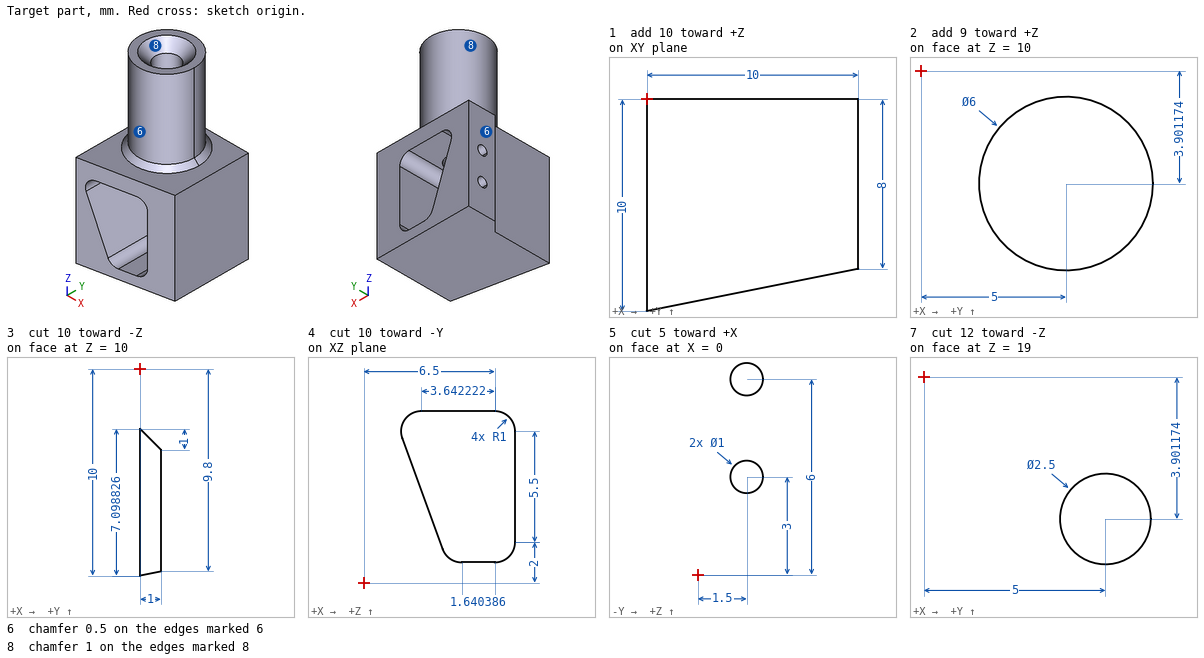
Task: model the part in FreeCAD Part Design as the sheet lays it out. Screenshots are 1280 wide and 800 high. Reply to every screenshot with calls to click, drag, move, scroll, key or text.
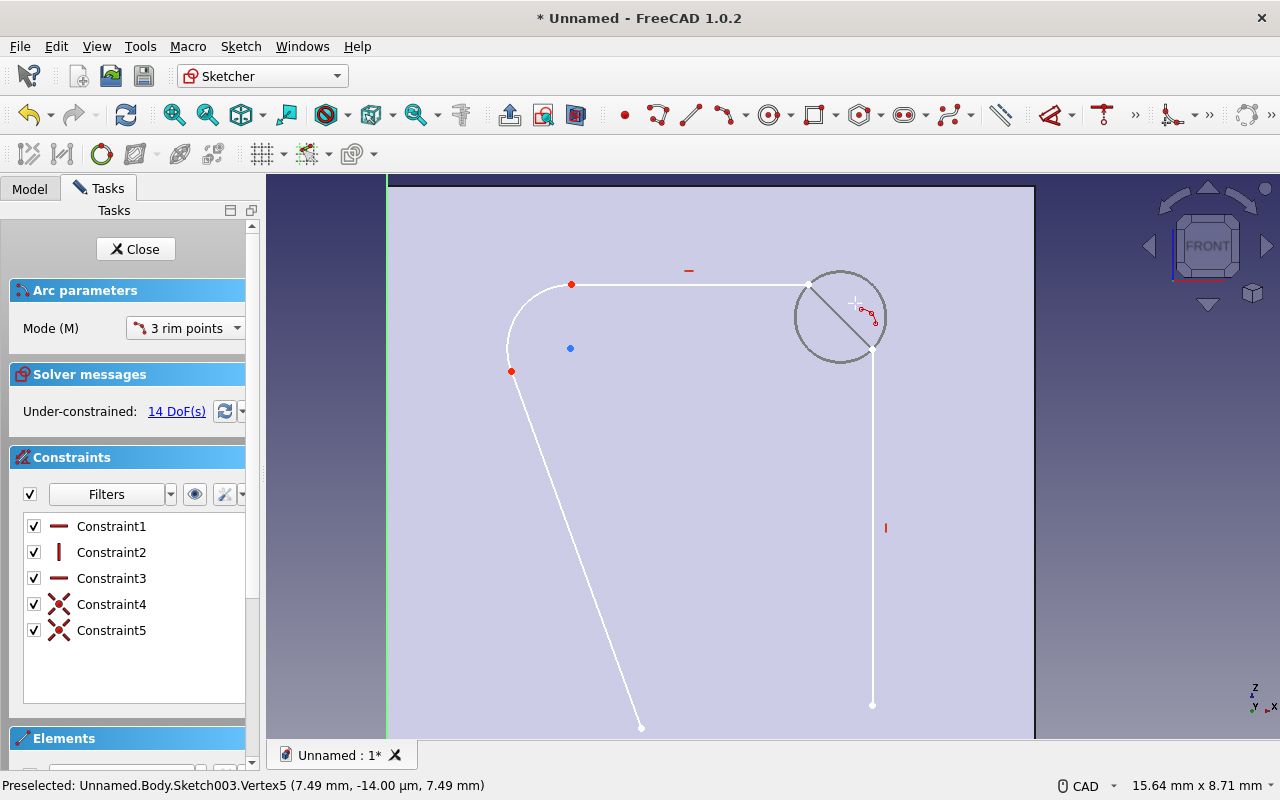
click(854, 302)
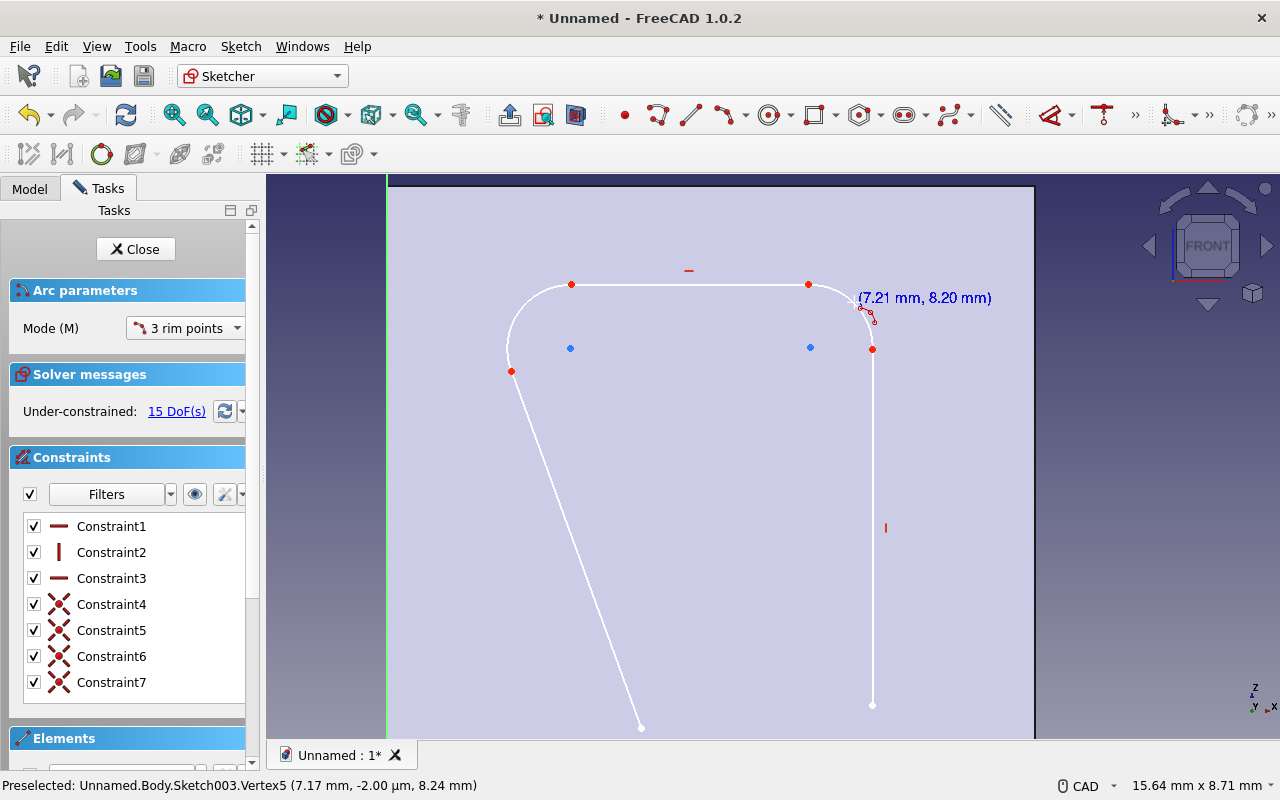
click(873, 706)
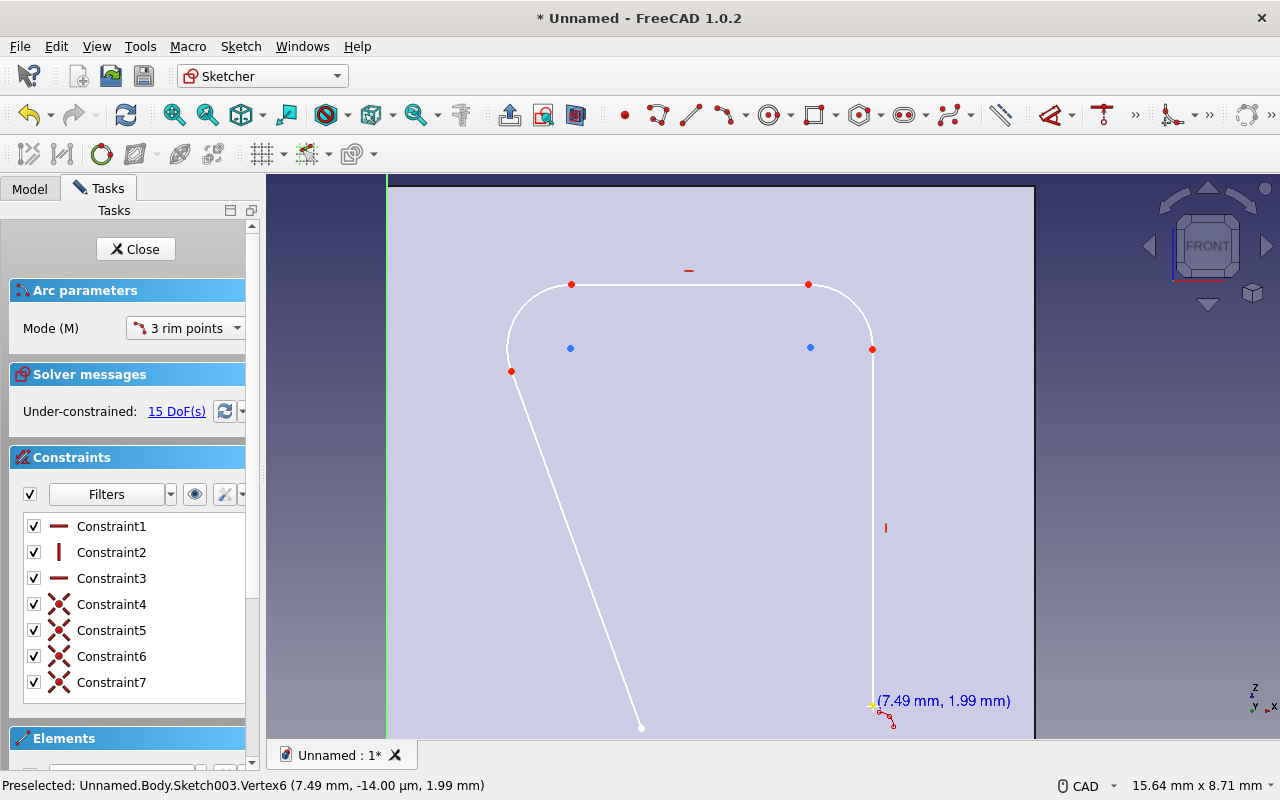
scroll(856, 248, down, 2)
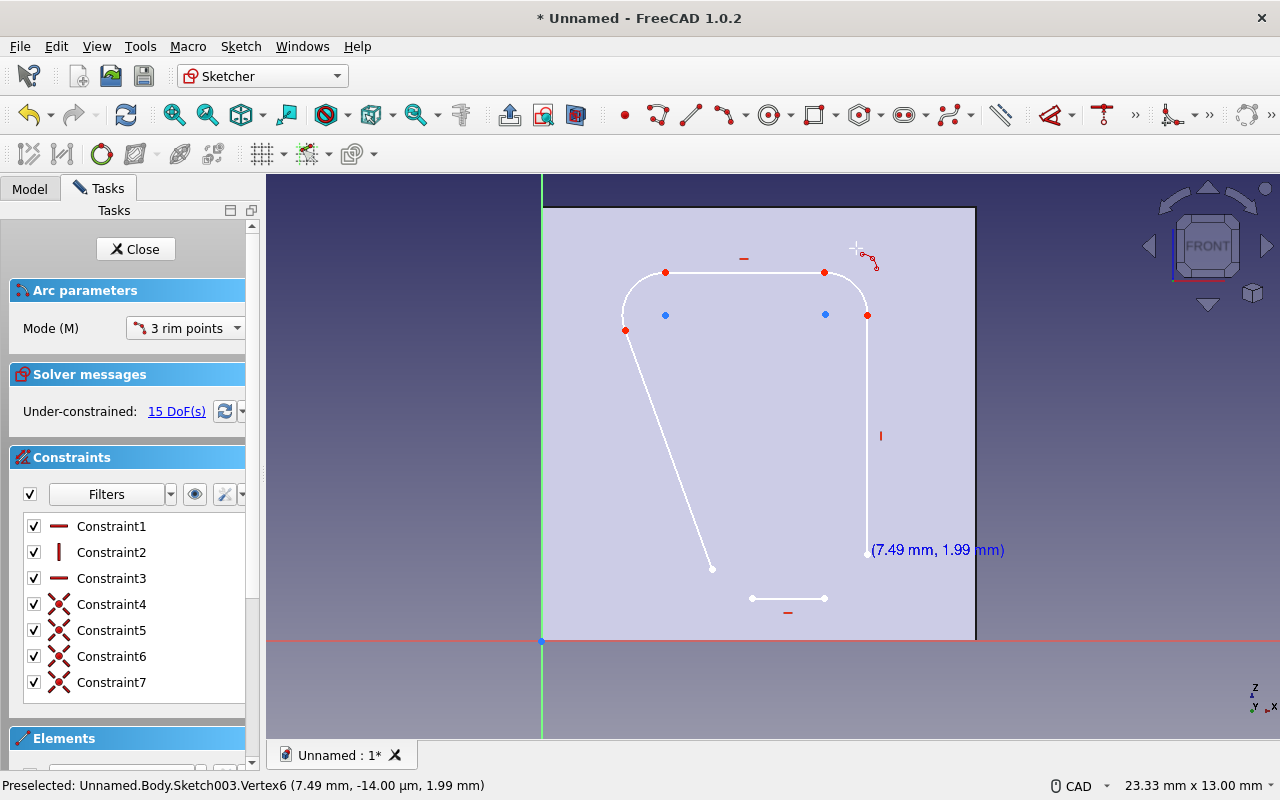
click(824, 599)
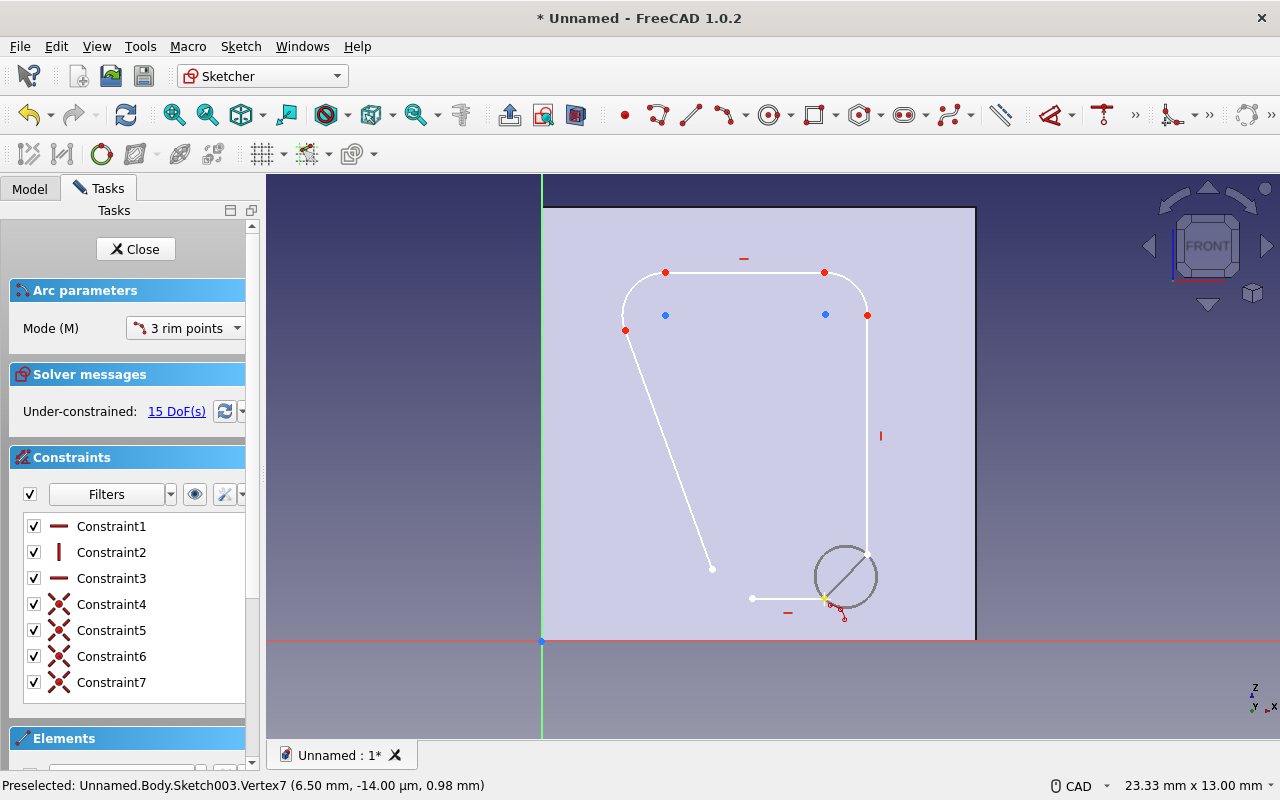
scroll(855, 585, up, 2)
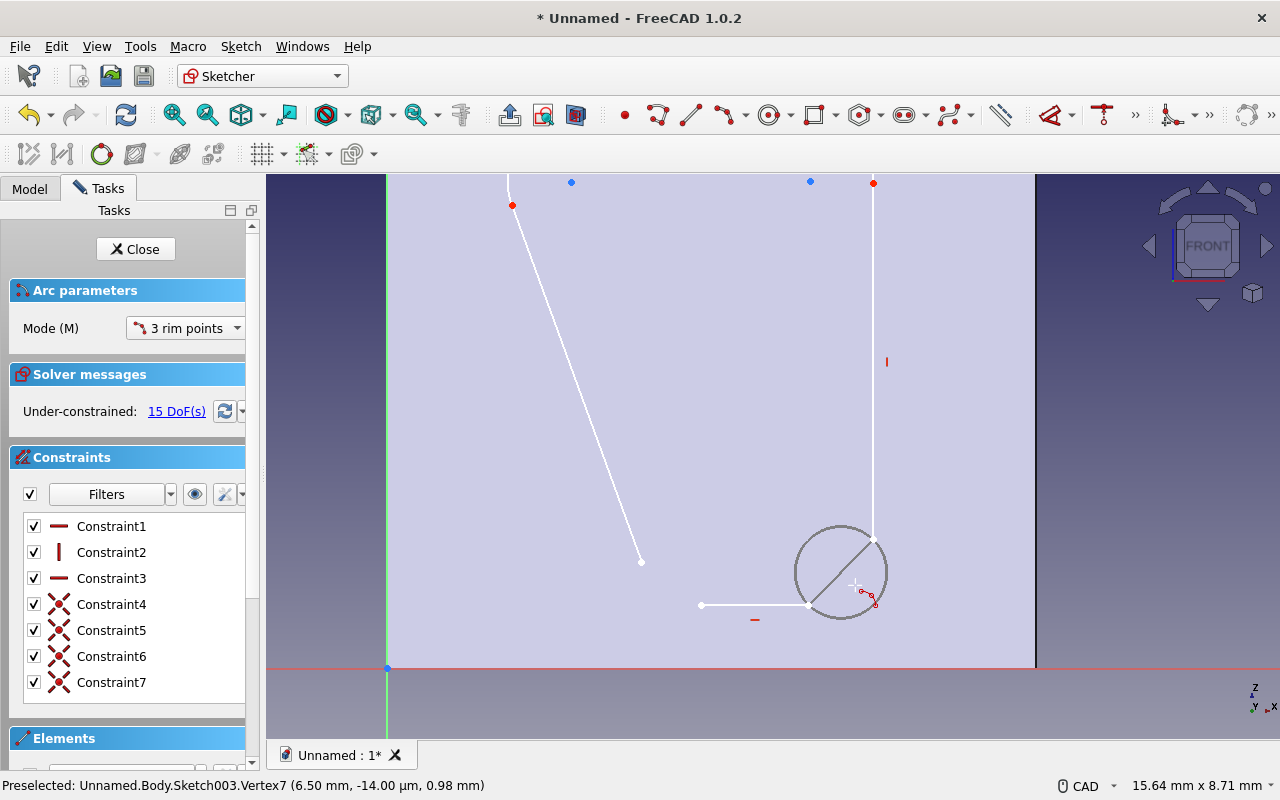
click(855, 585)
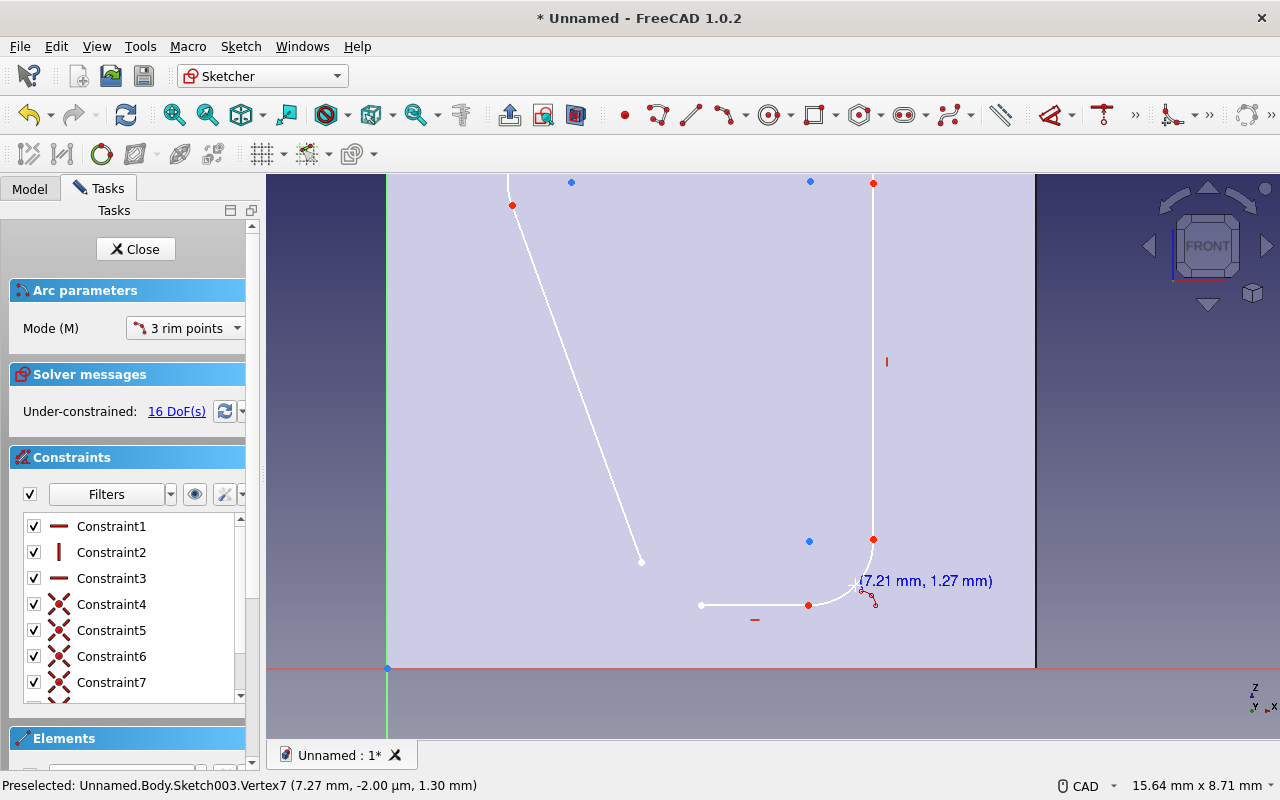
click(702, 605)
click(642, 562)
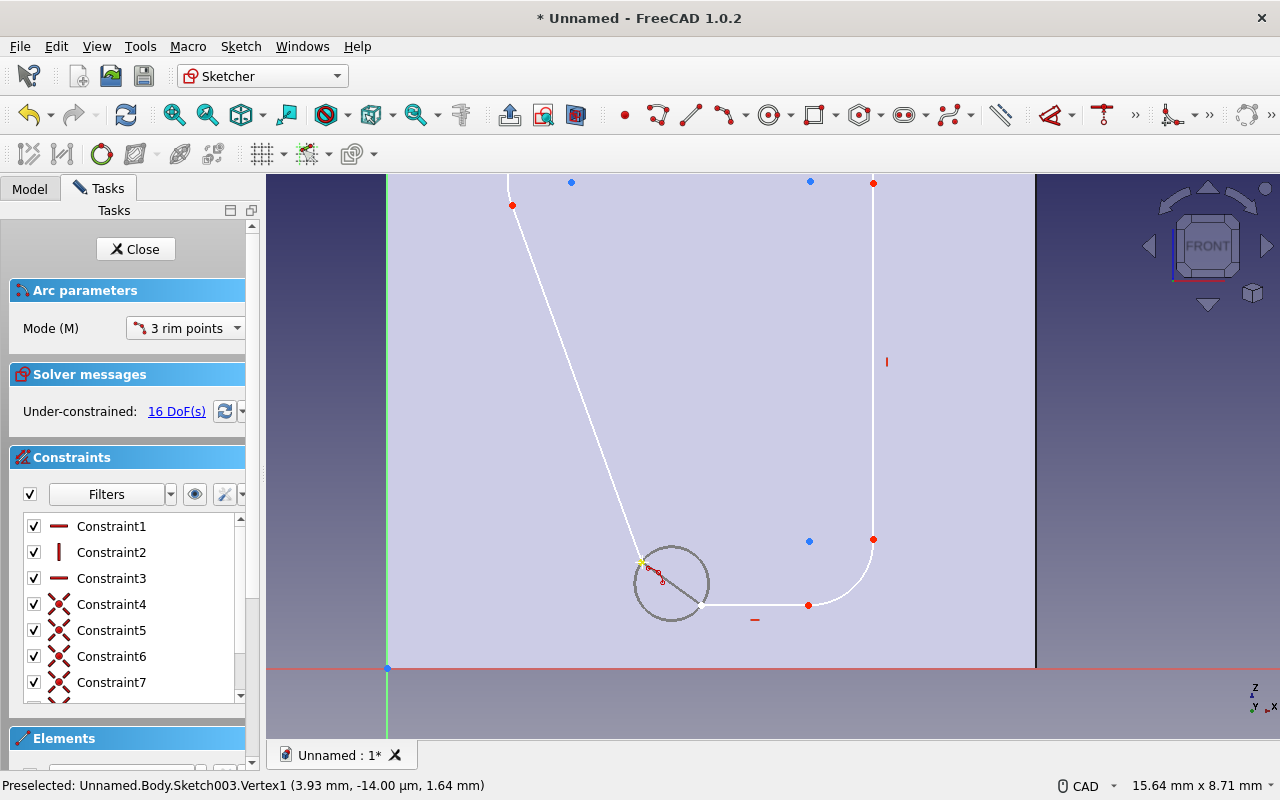
scroll(665, 592, up, 2)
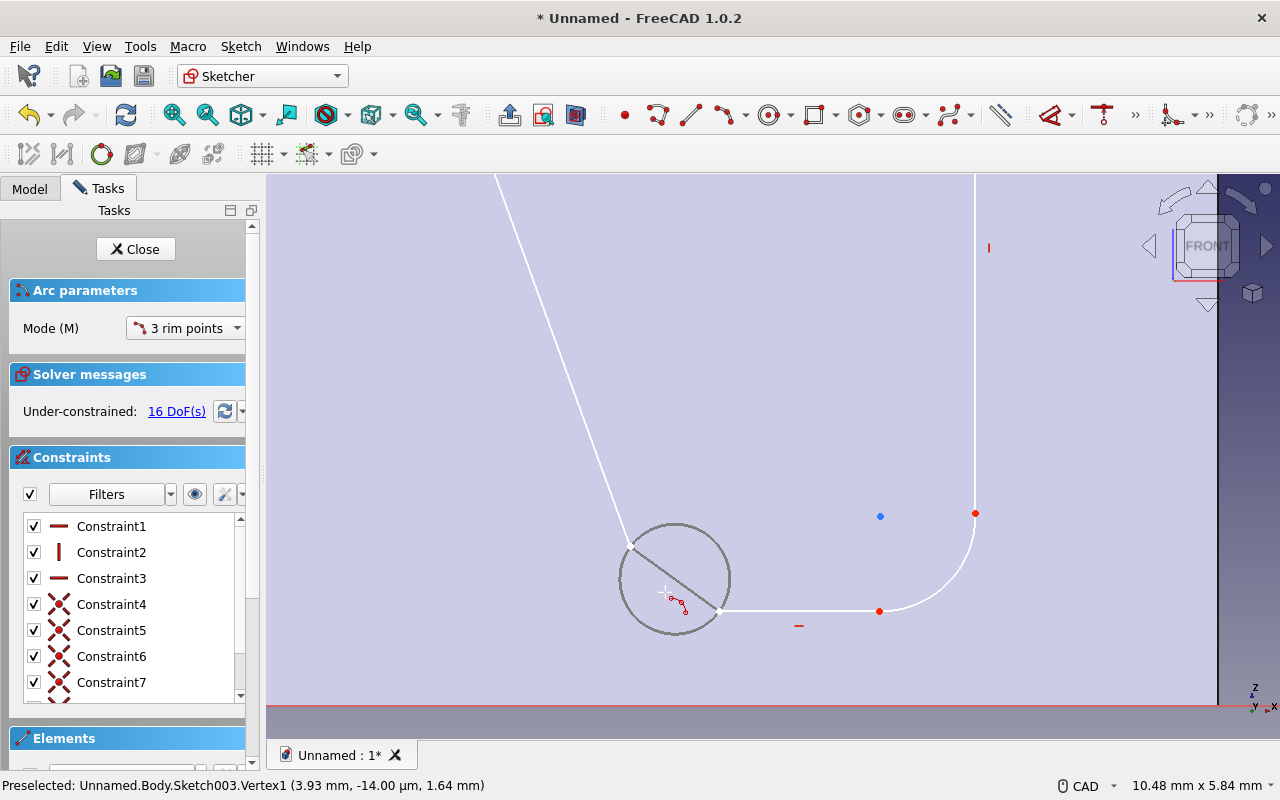
click(665, 592)
key(Escape)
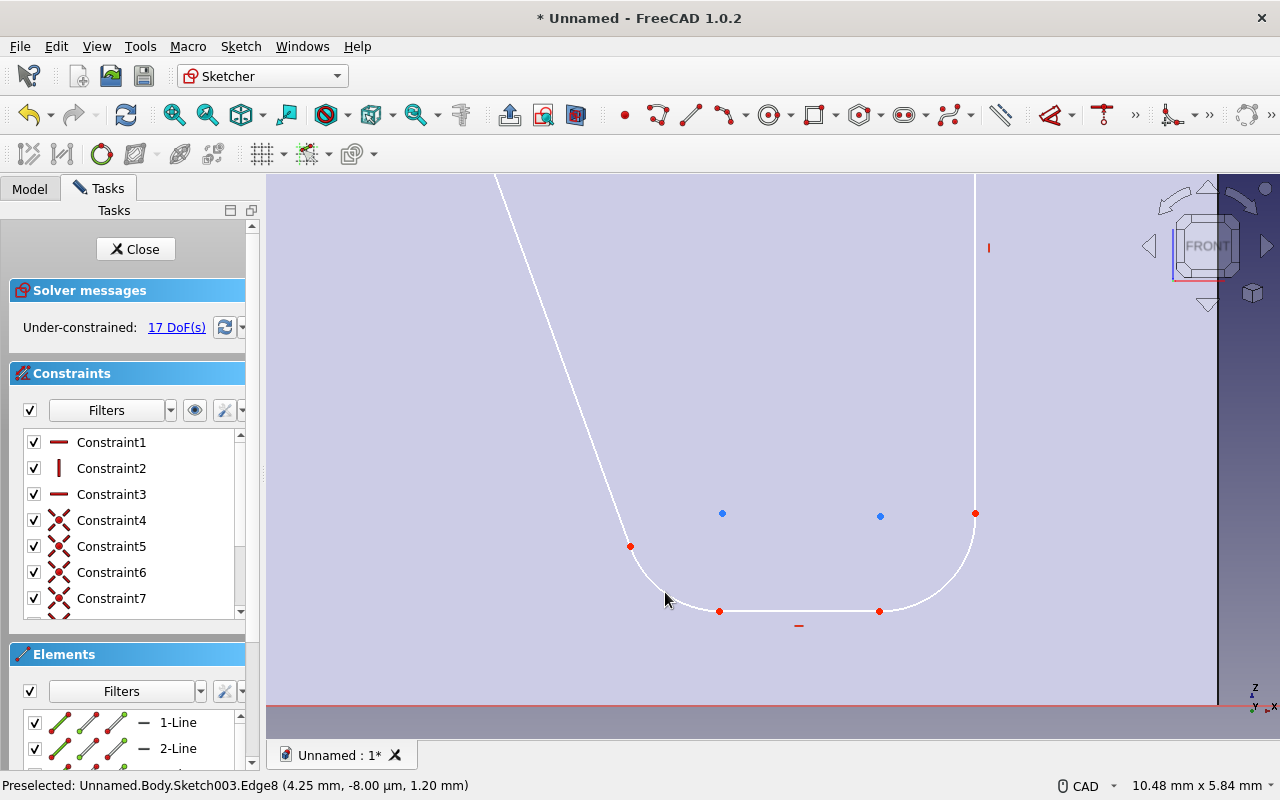
click(572, 387)